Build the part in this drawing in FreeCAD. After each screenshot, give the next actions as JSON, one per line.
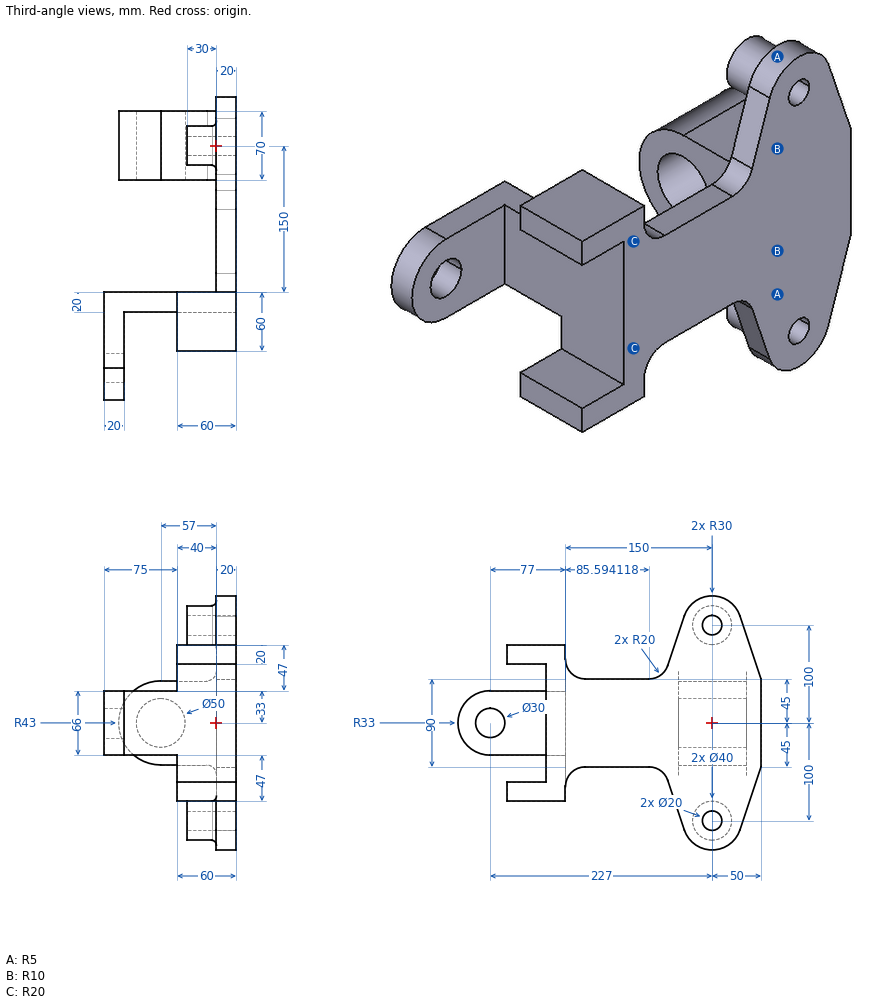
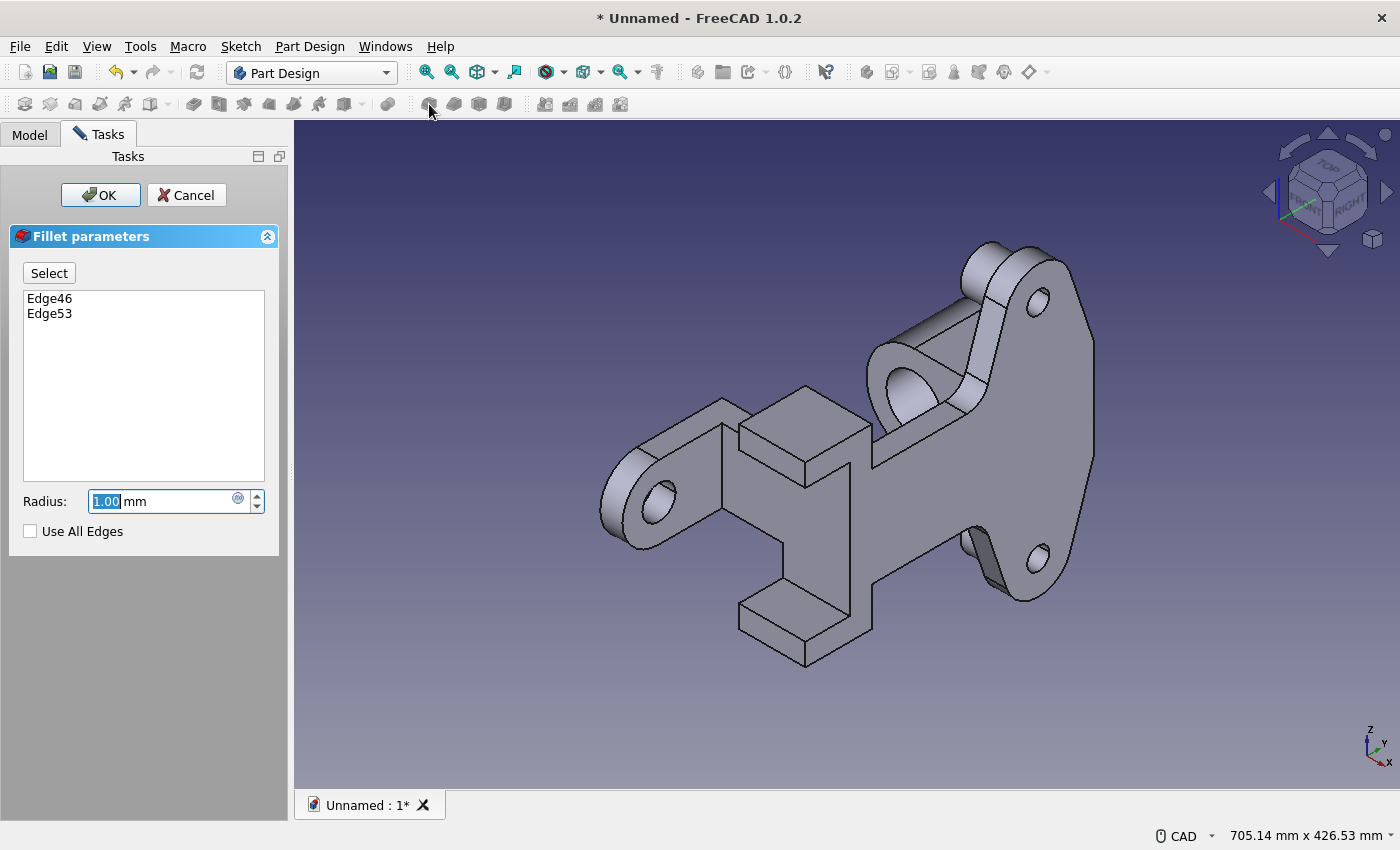
{"action": "type", "text": "20"}
{"action": "key", "text": "Tab"}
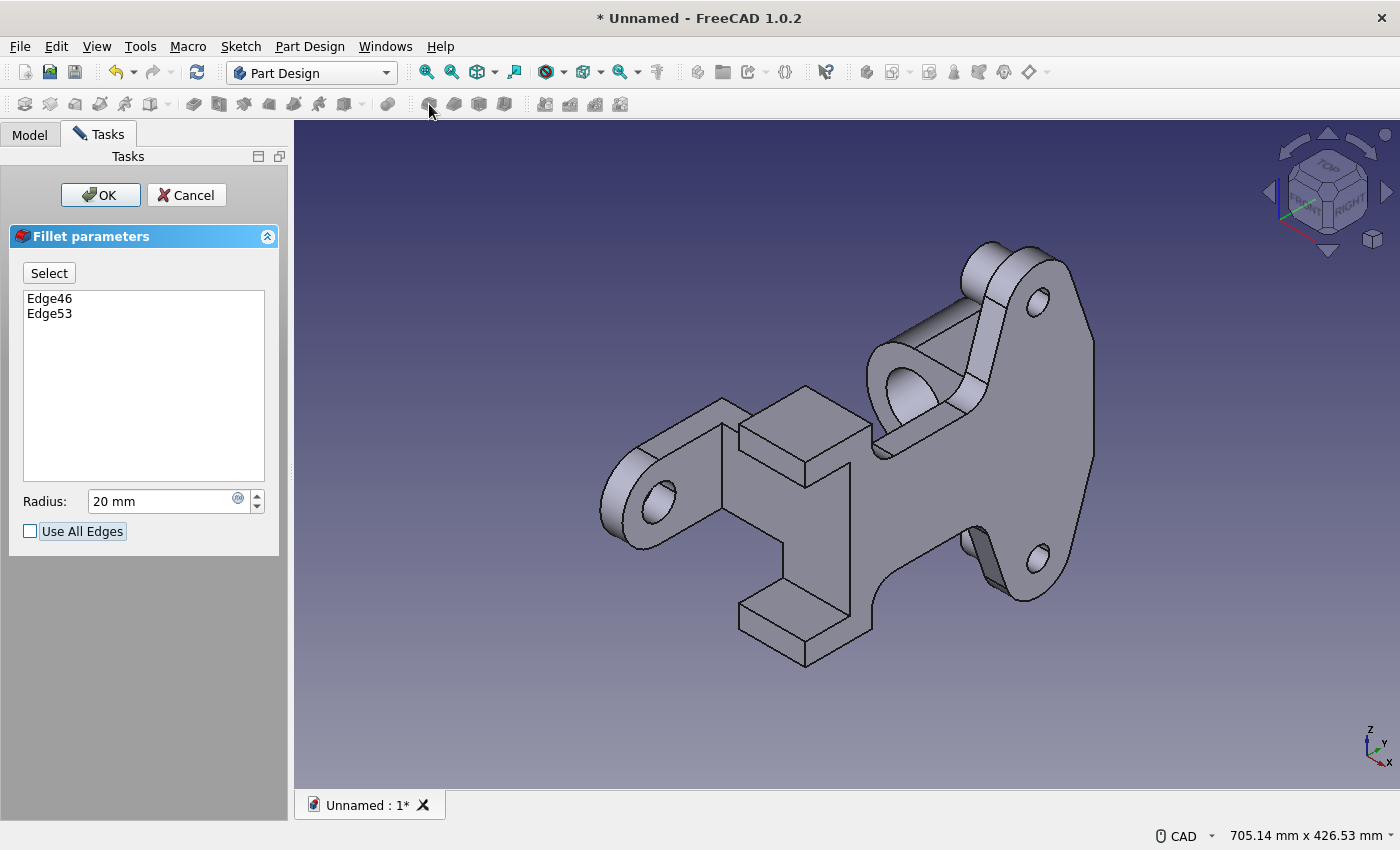
{"action": "left_click", "coordinate": [101, 195]}